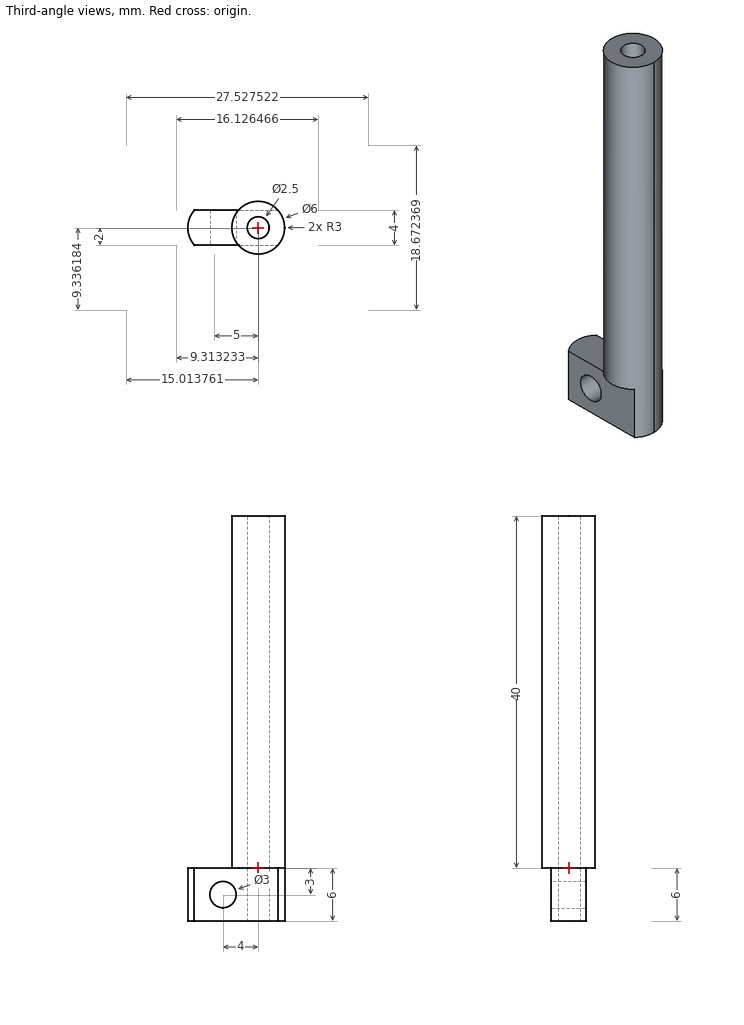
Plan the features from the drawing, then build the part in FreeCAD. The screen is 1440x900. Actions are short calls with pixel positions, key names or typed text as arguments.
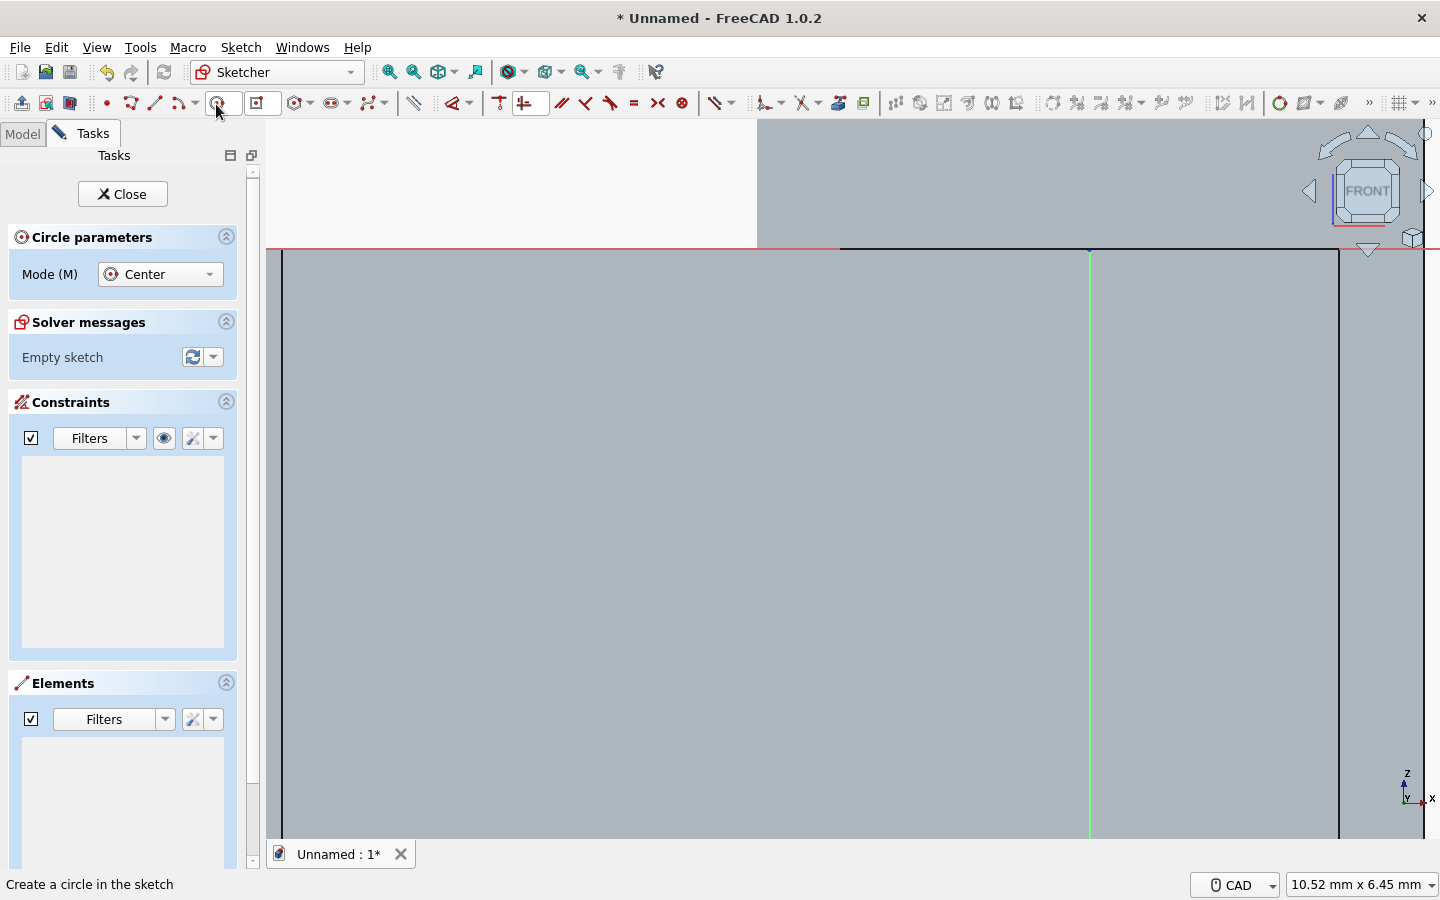
click(643, 584)
move(761, 465)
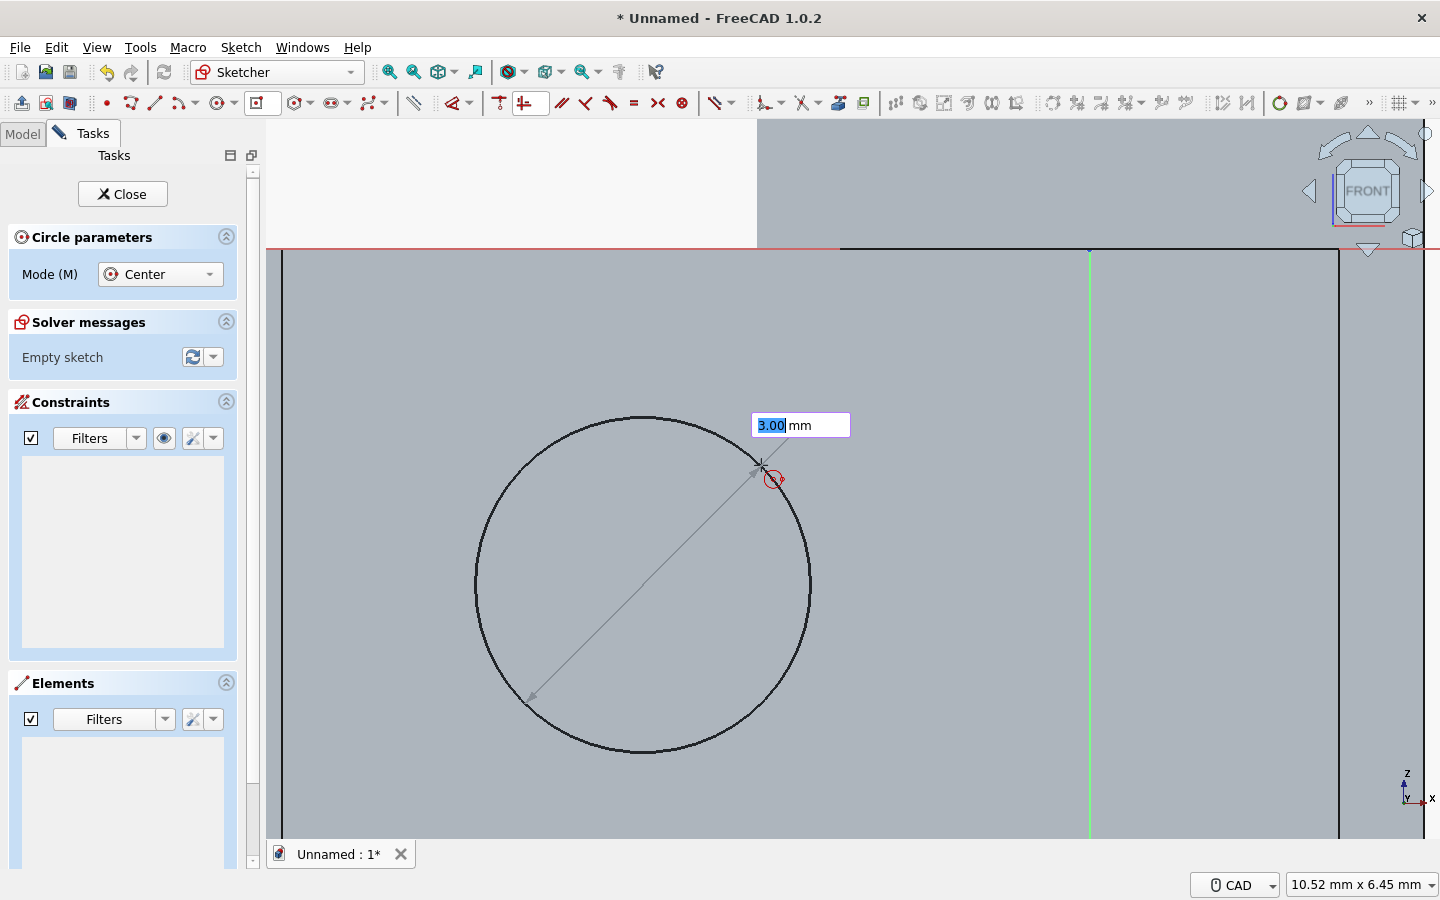
text(3)
key(Return)
key(Escape)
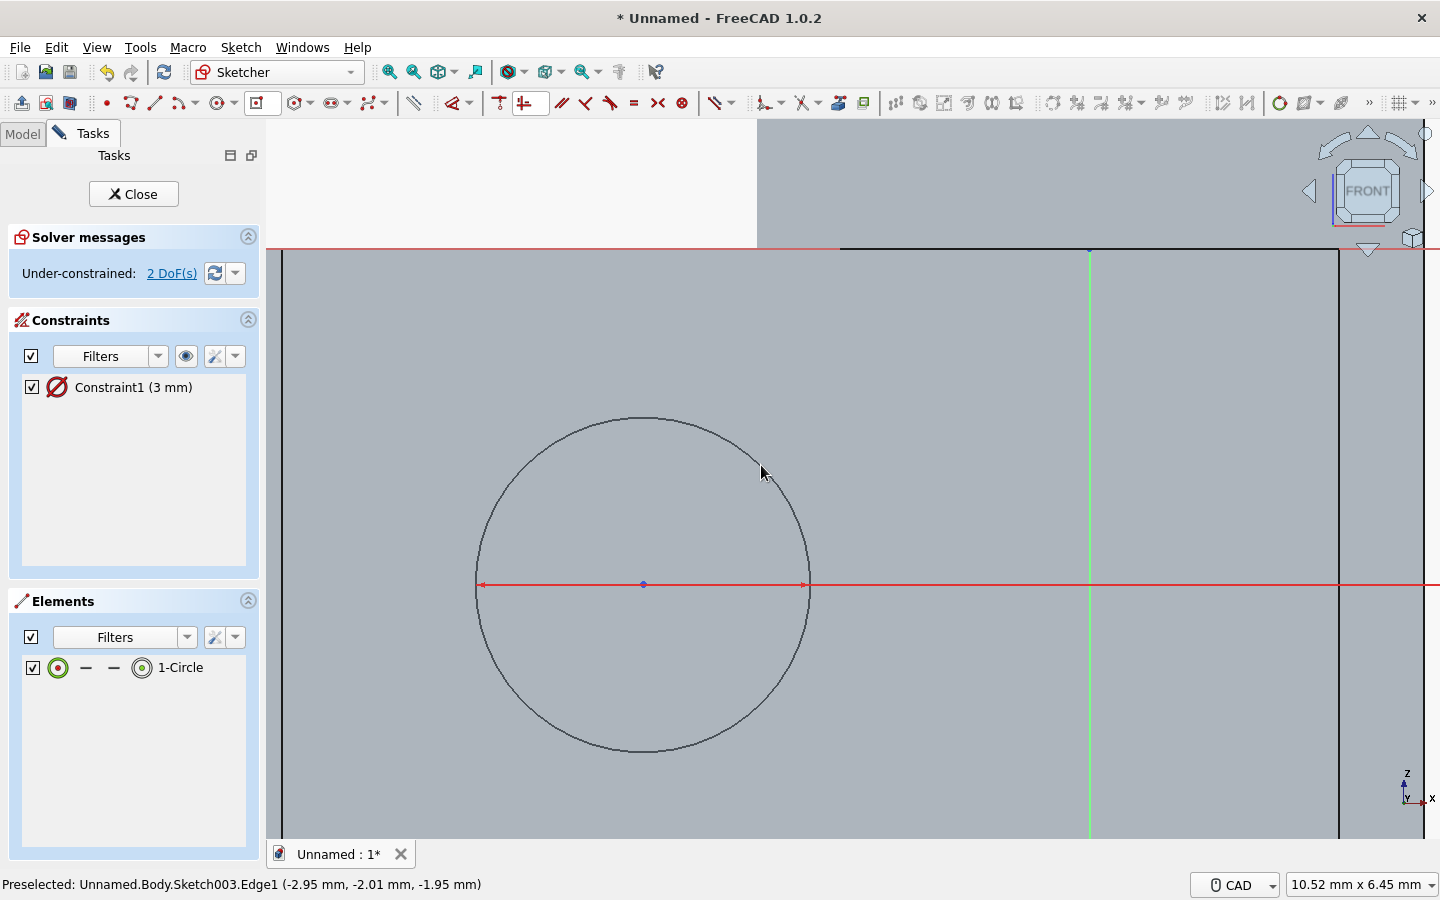
click(452, 104)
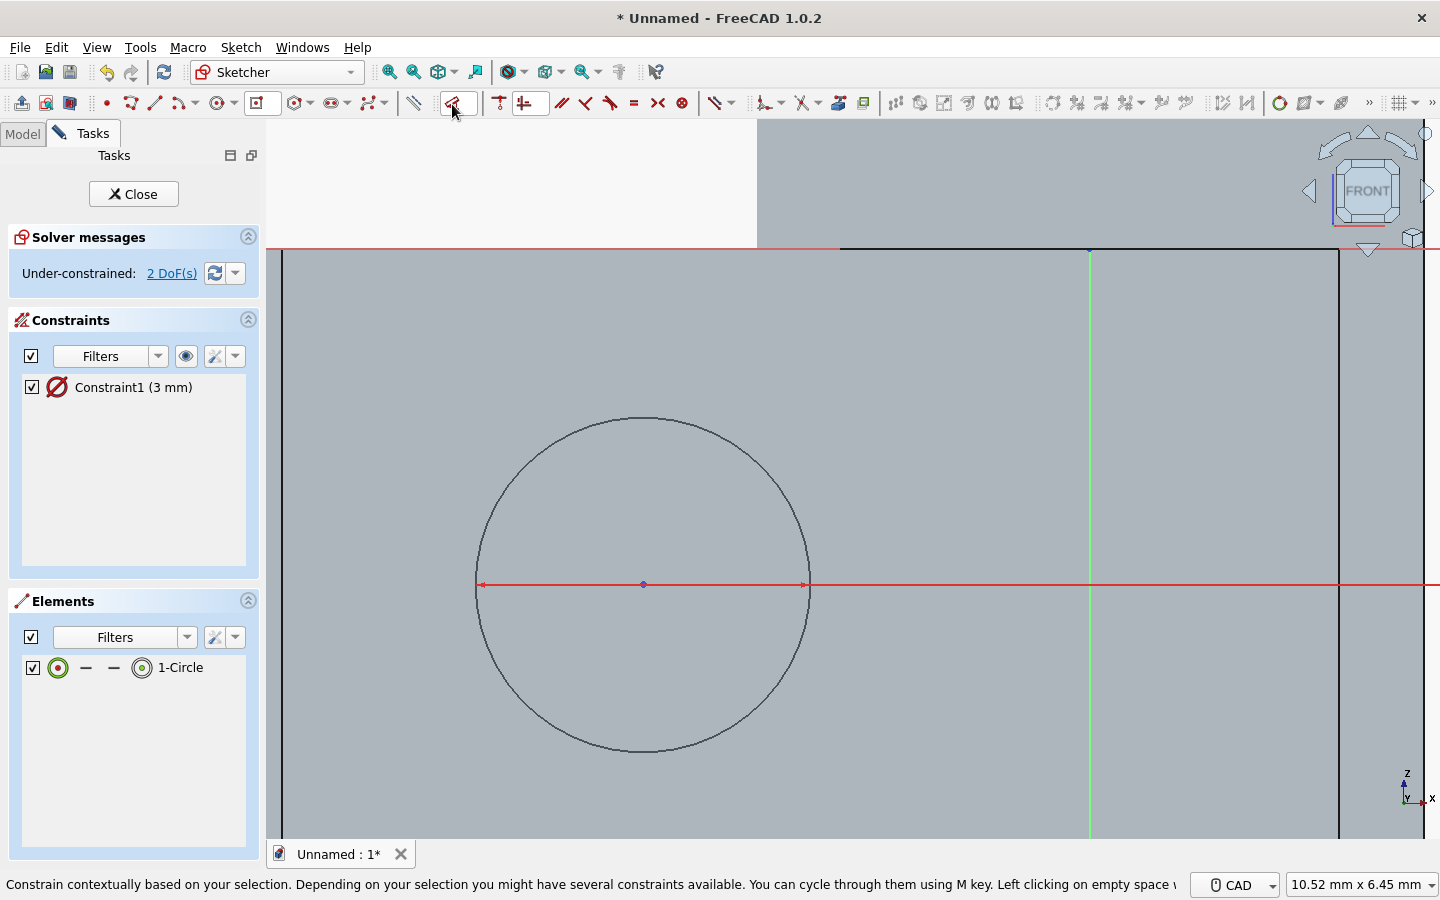
click(643, 585)
click(866, 215)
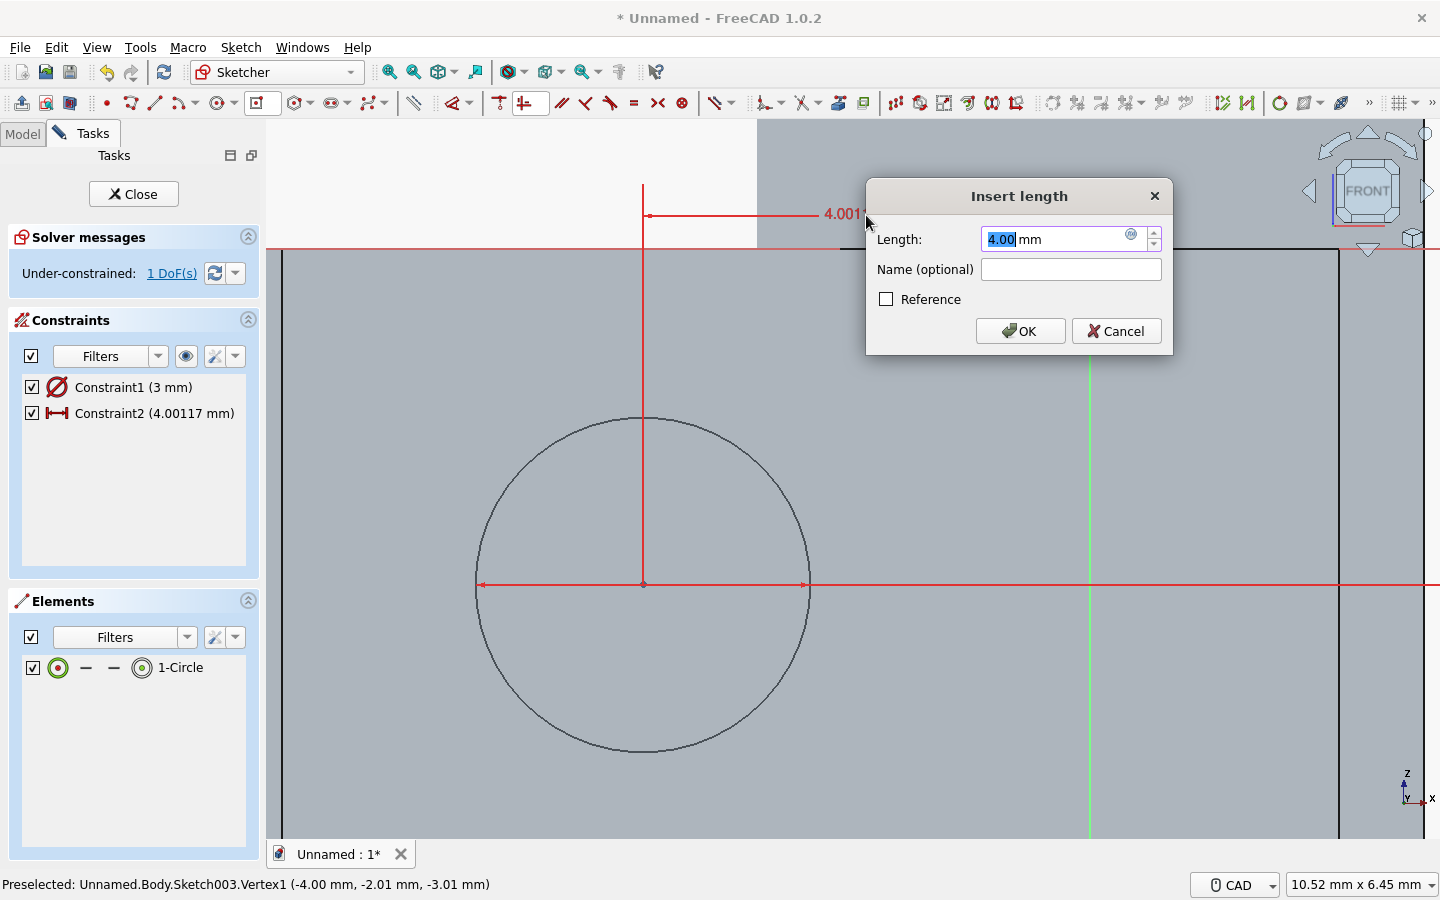
text(4)
key(Return)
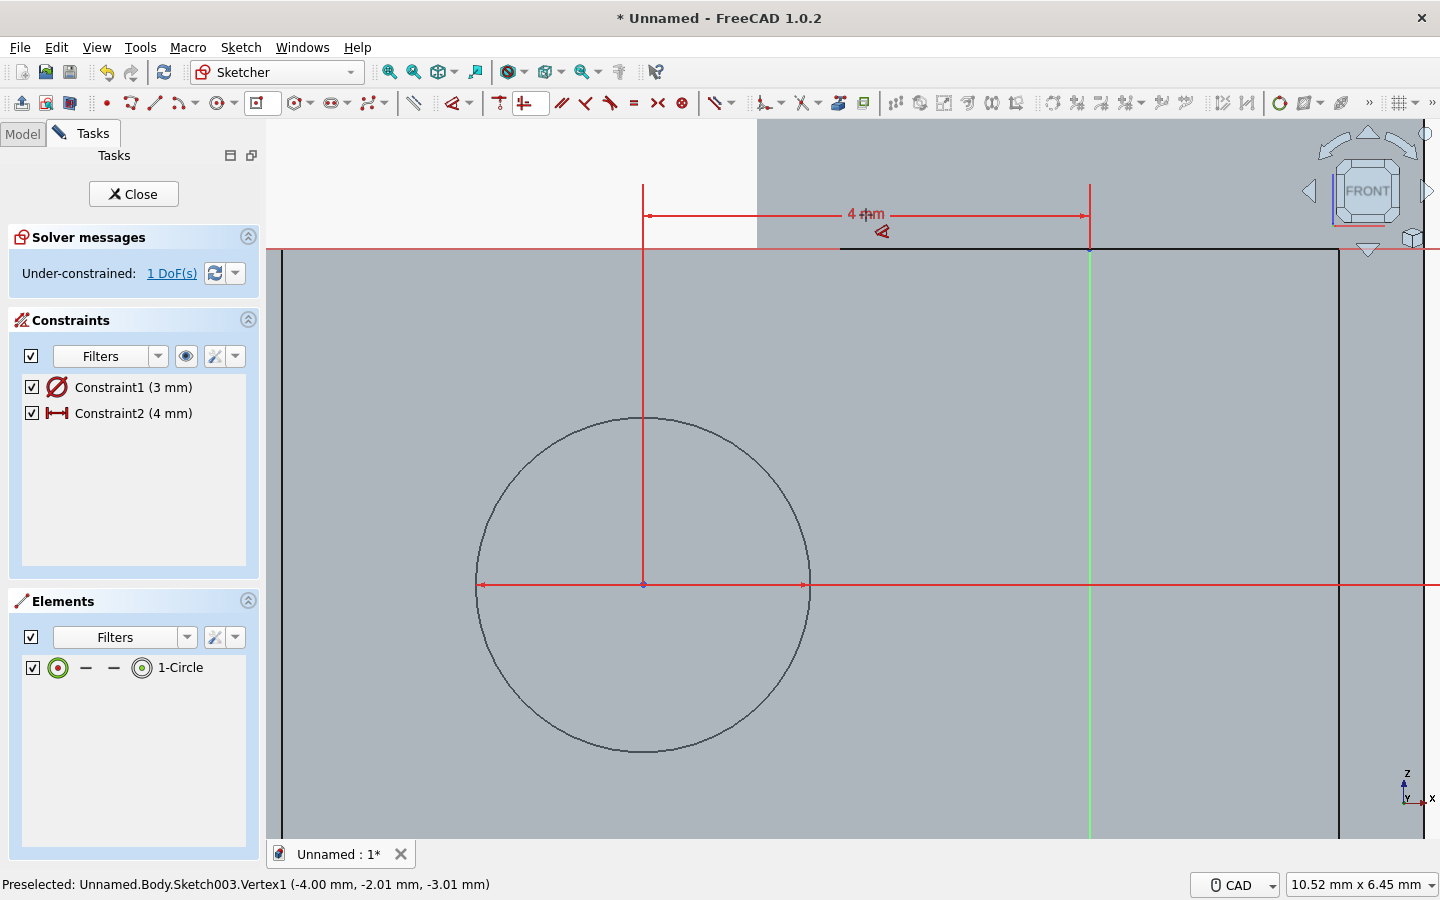
click(643, 585)
click(1124, 417)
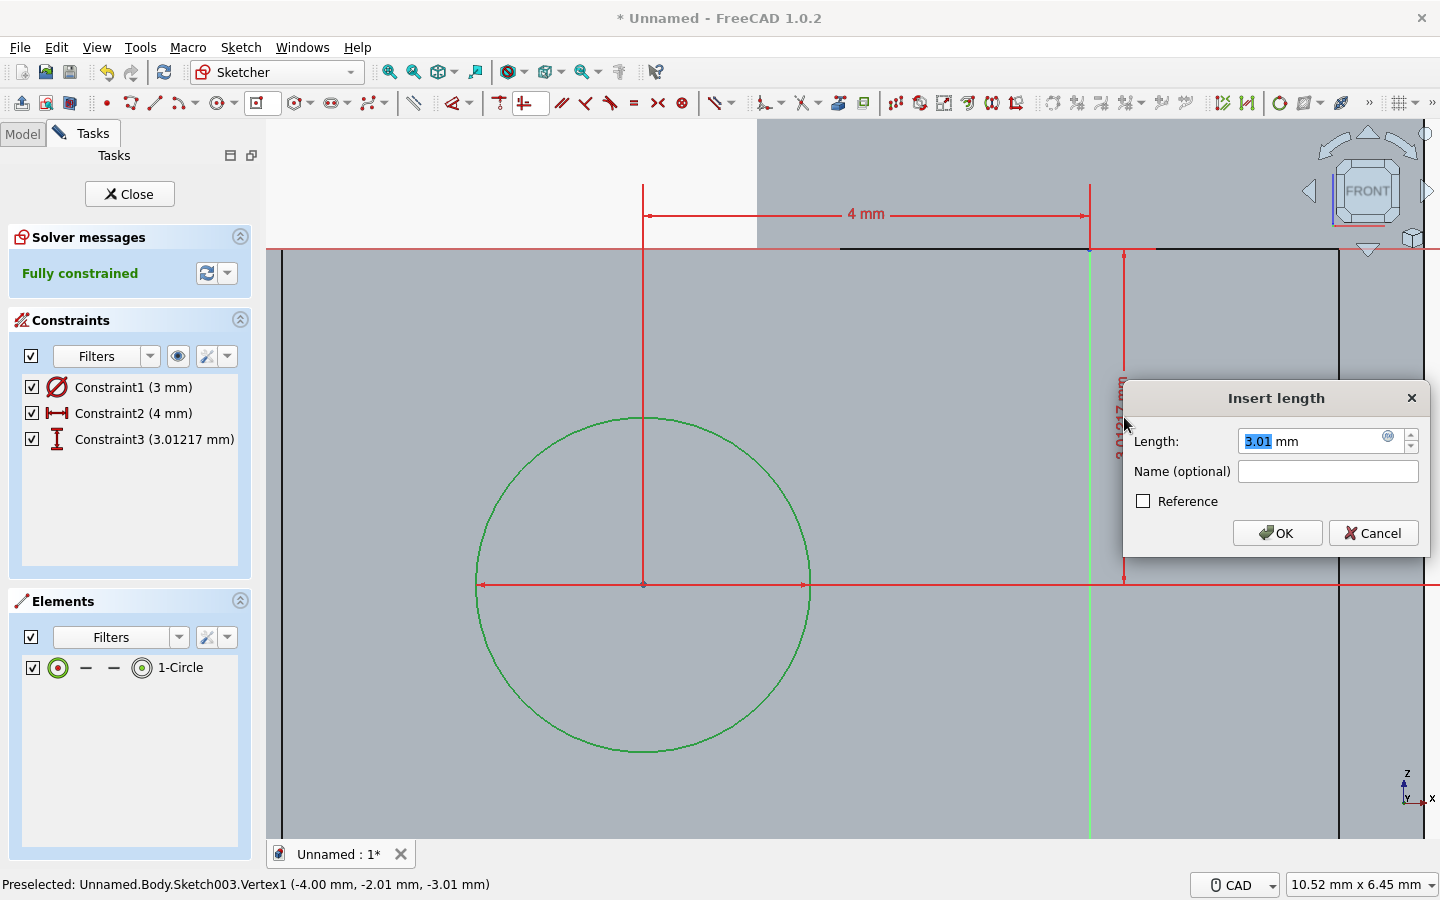
text(3)
key(Return)
key(Escape)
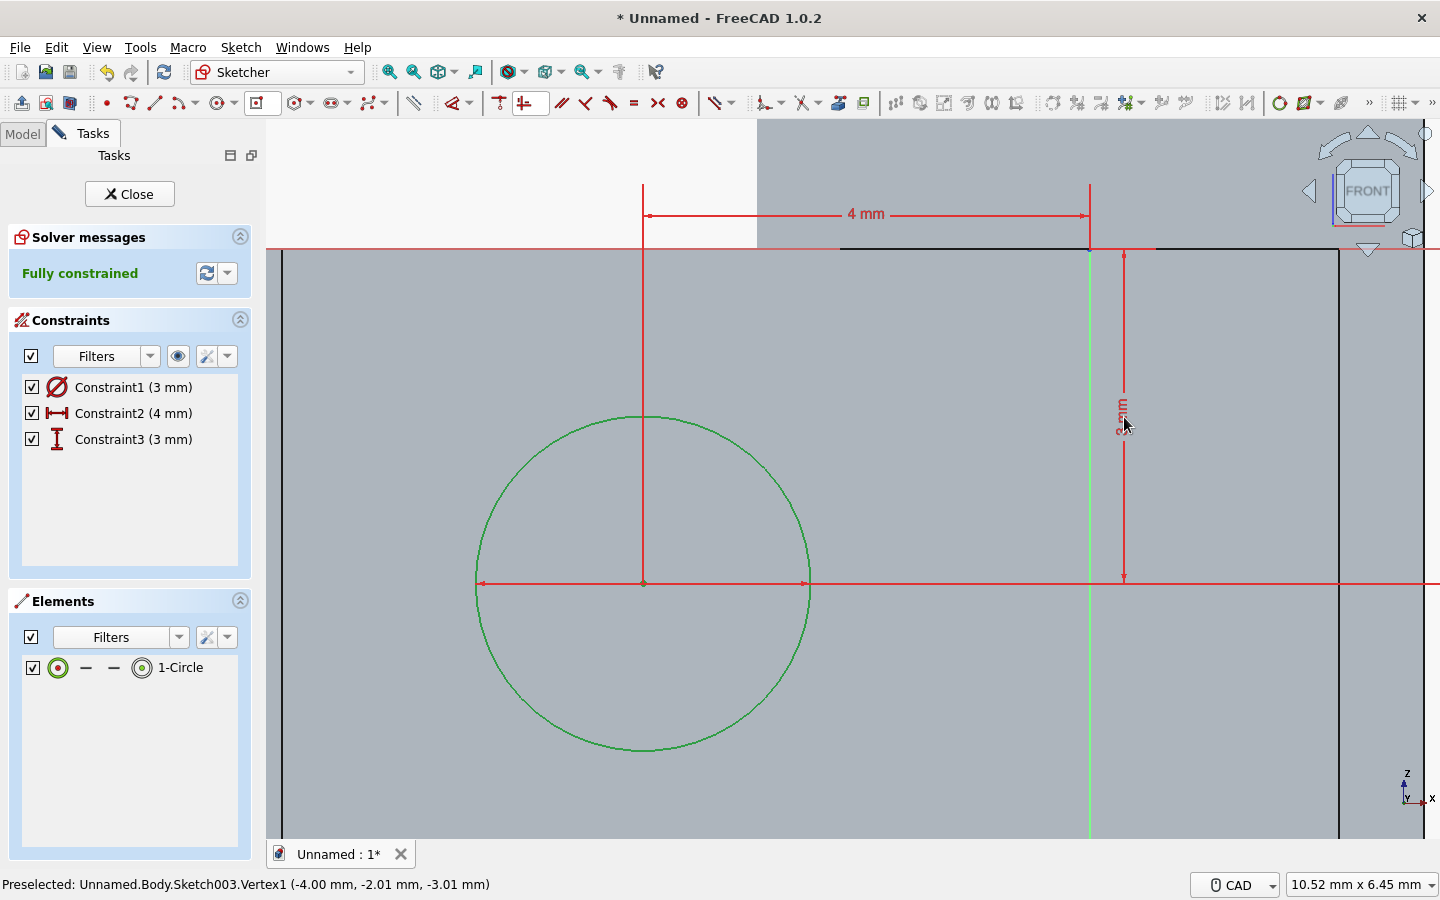
click(130, 194)